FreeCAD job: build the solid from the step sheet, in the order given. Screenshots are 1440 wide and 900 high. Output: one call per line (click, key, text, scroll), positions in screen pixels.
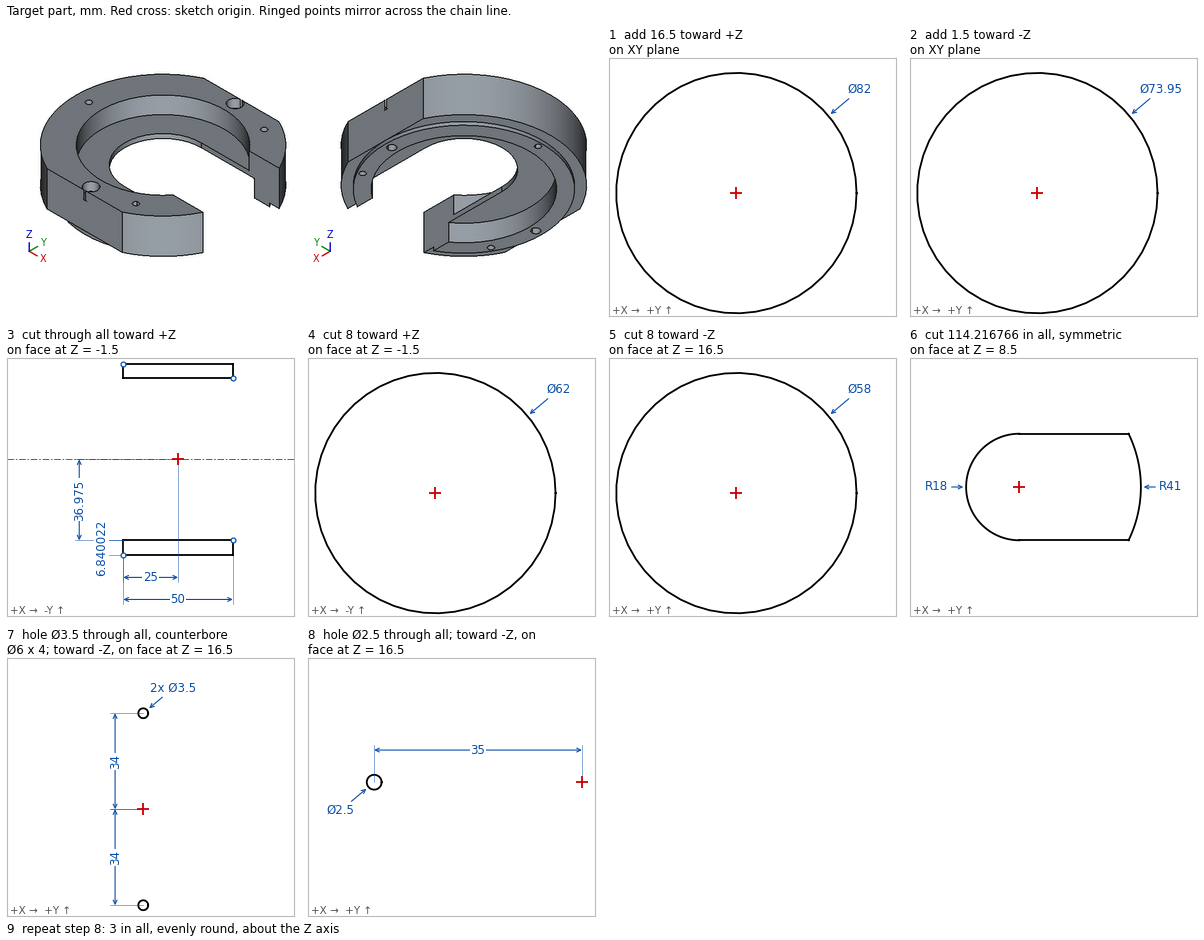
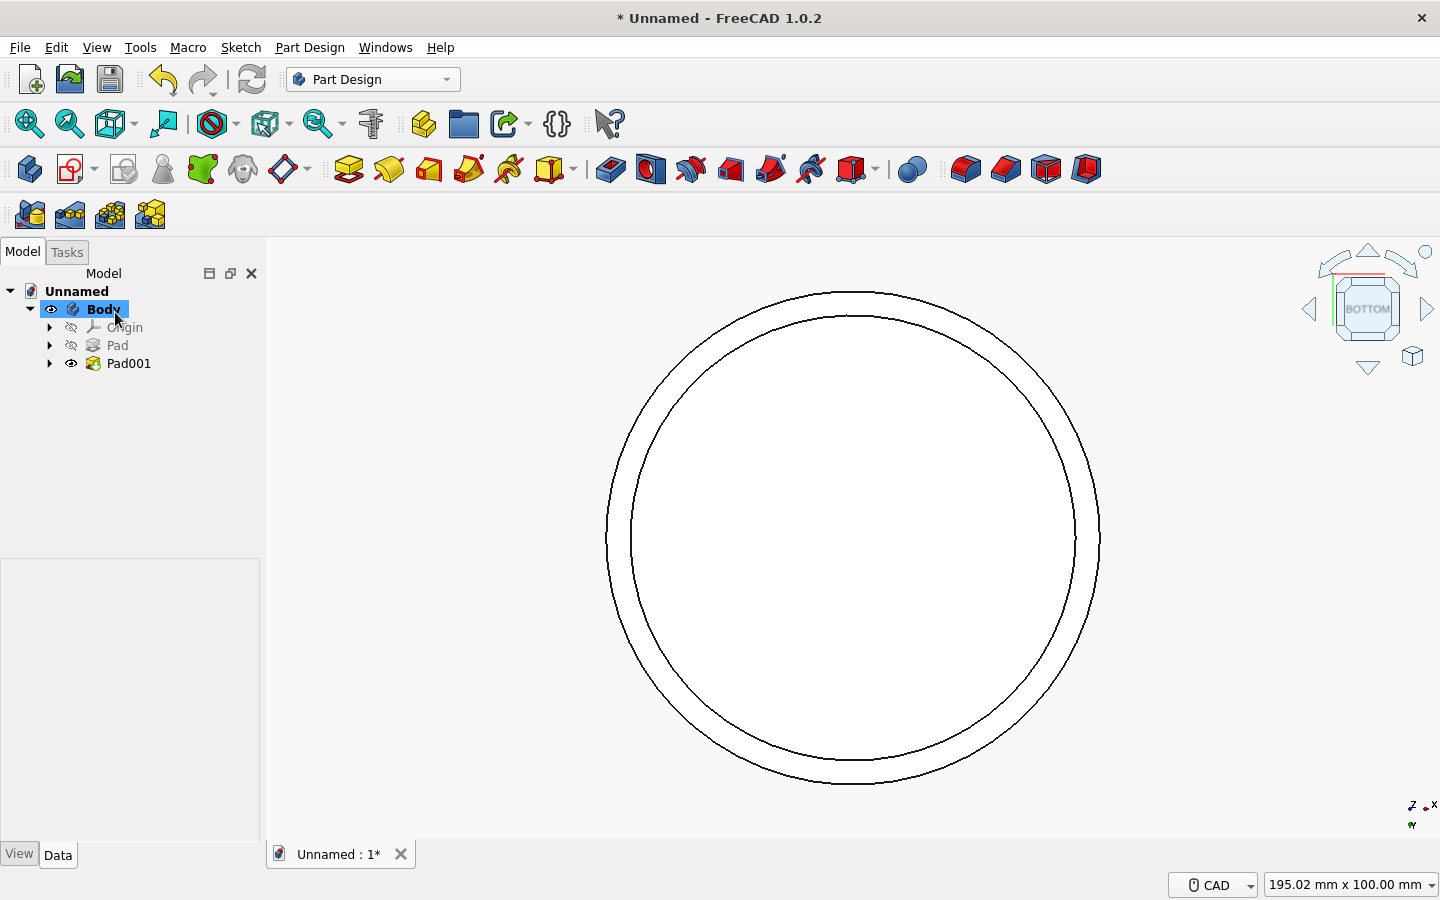
click(853, 537)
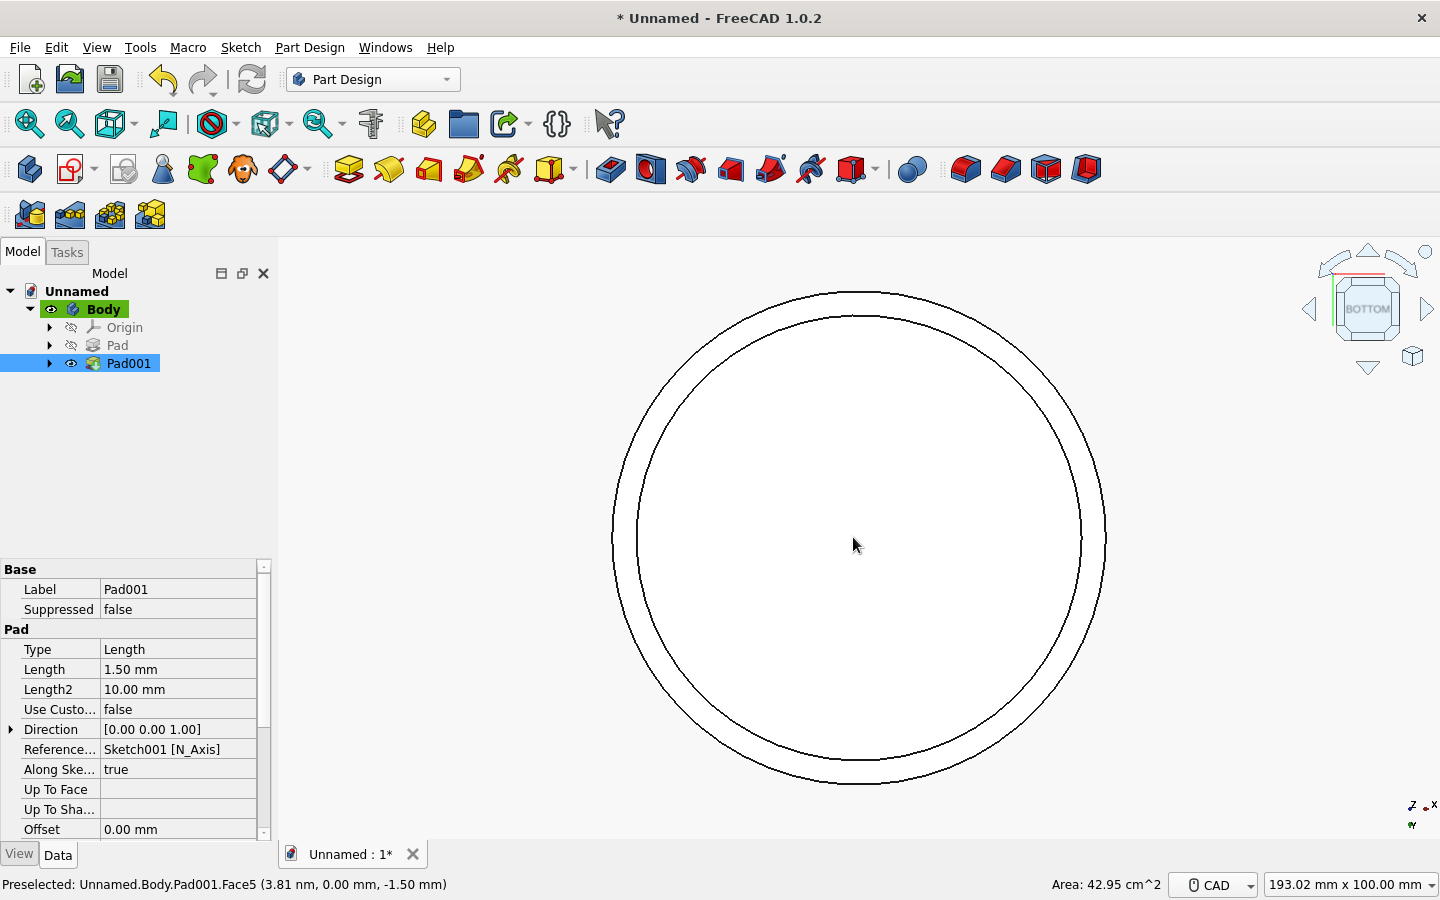
click(70, 170)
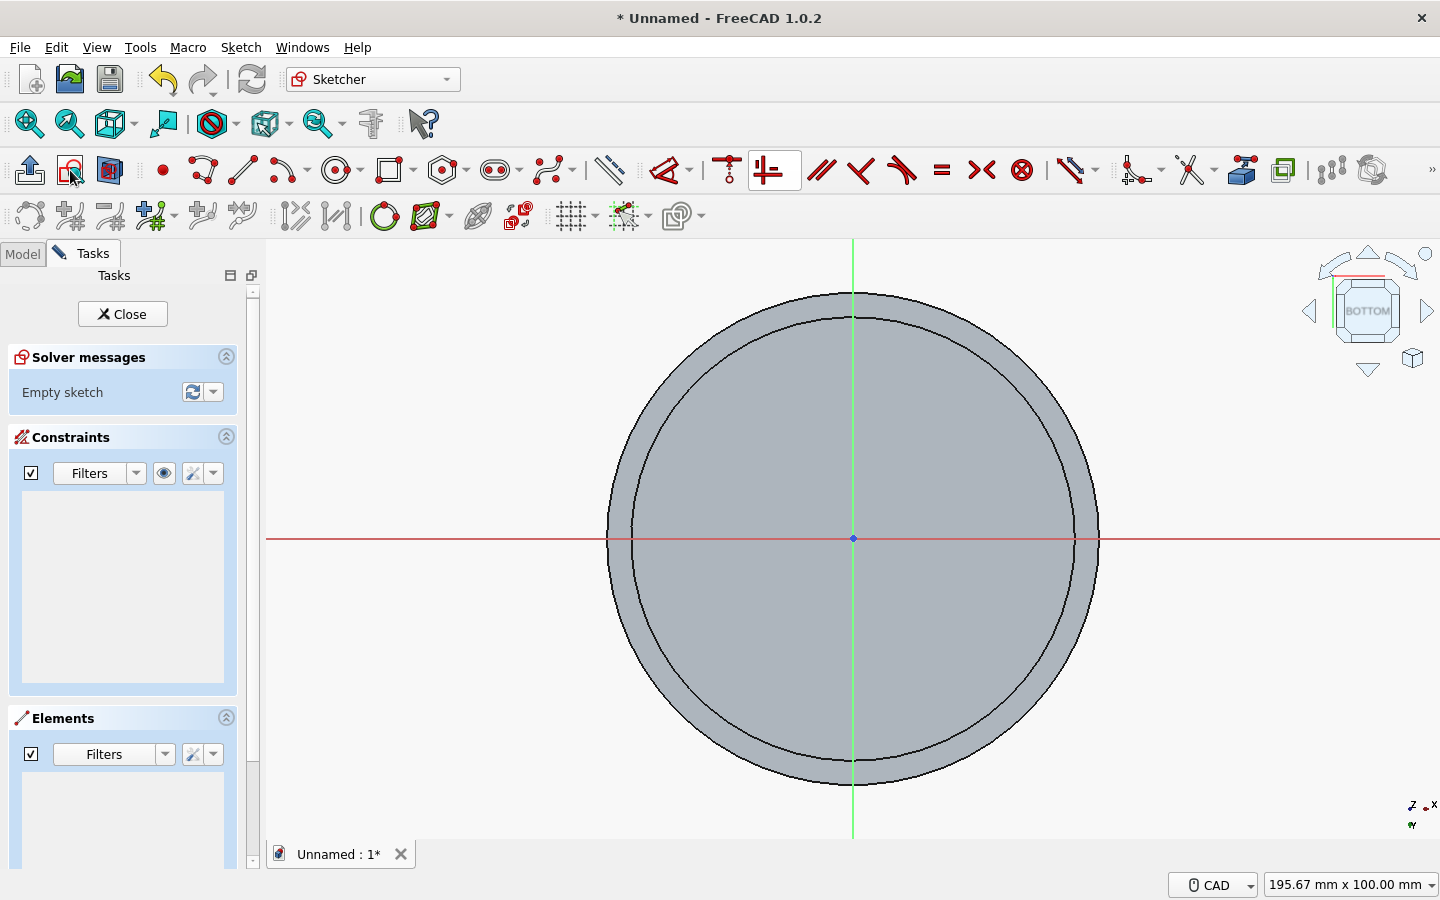
scroll(645, 539, down, 2)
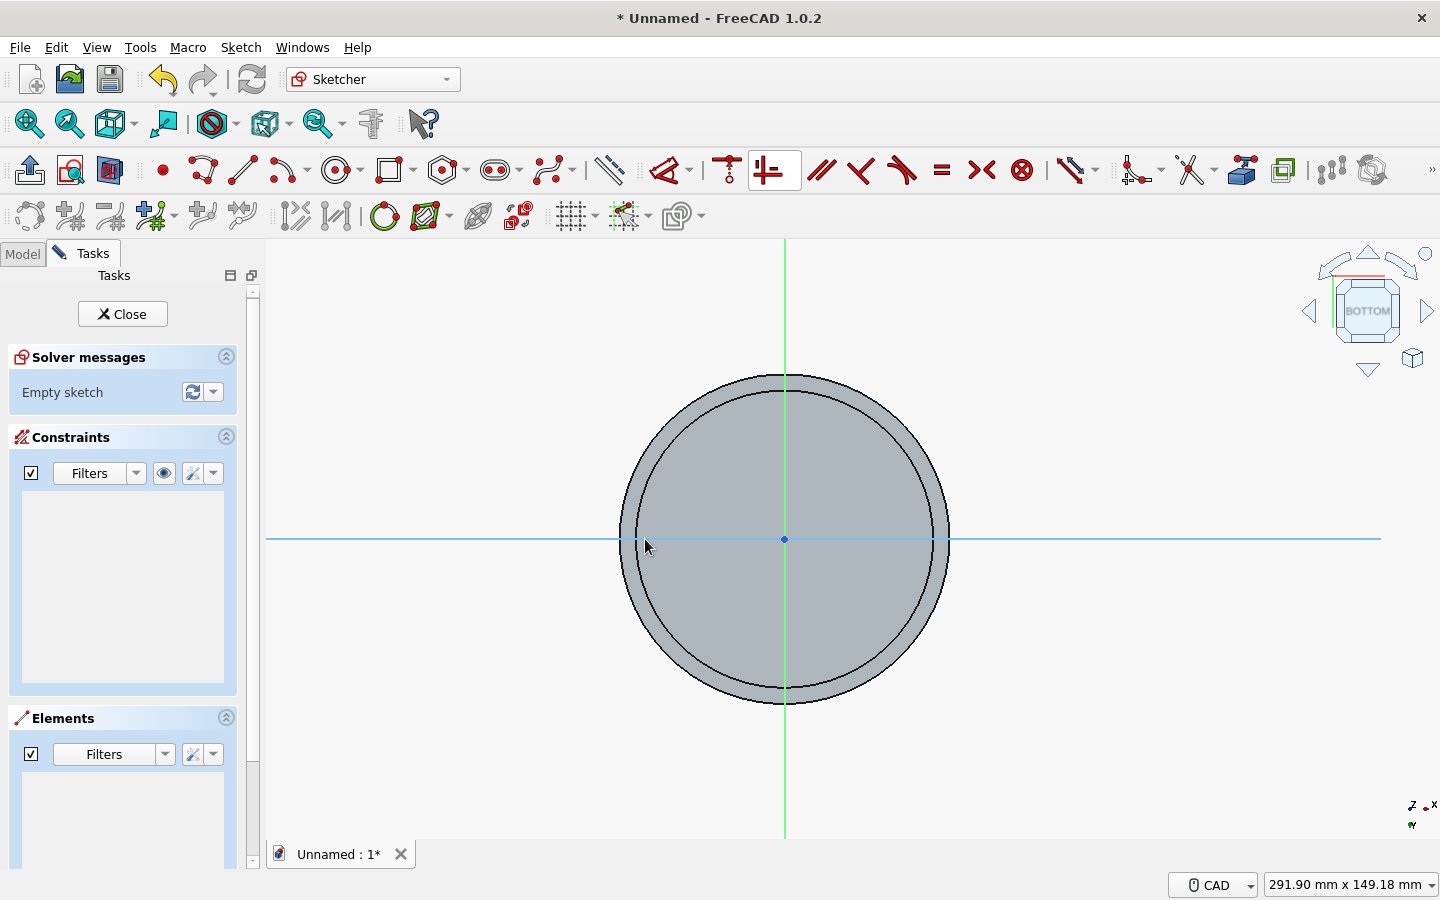
key(g)
key(r)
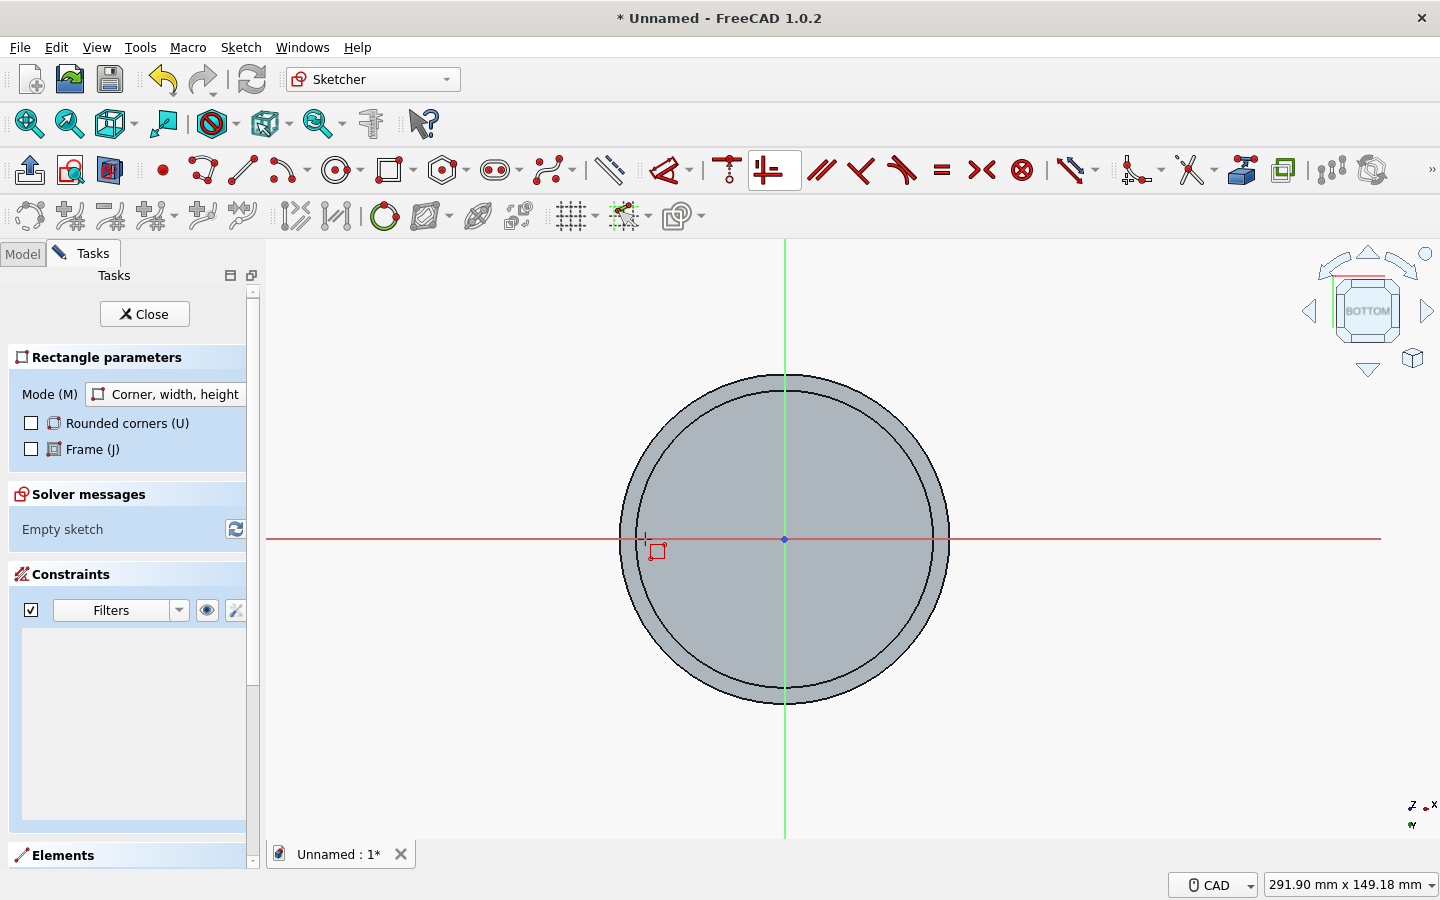
click(684, 688)
click(885, 715)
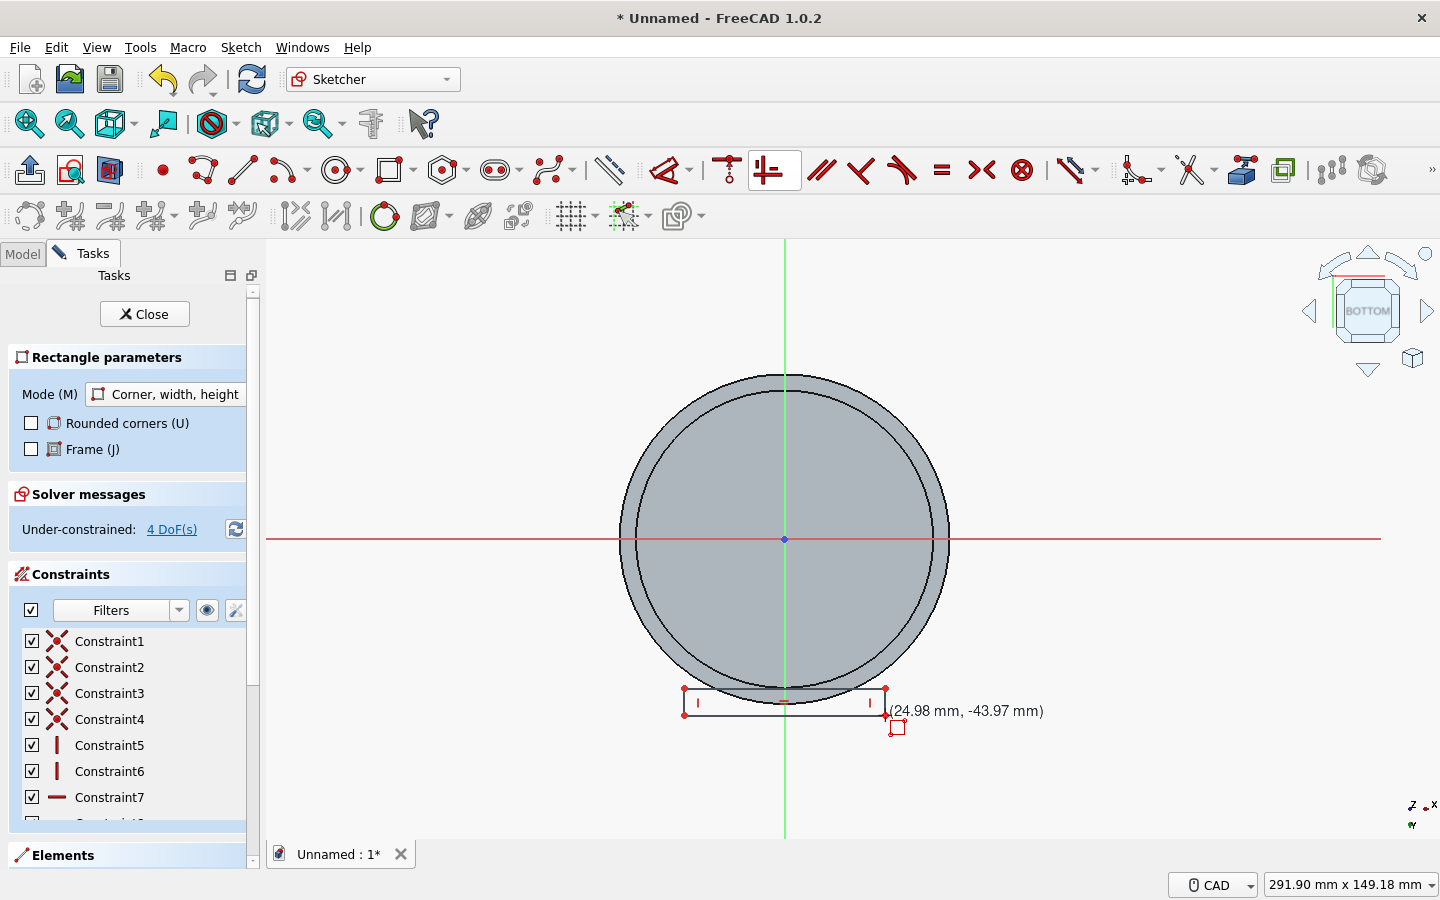
click(684, 363)
click(885, 390)
key(Escape)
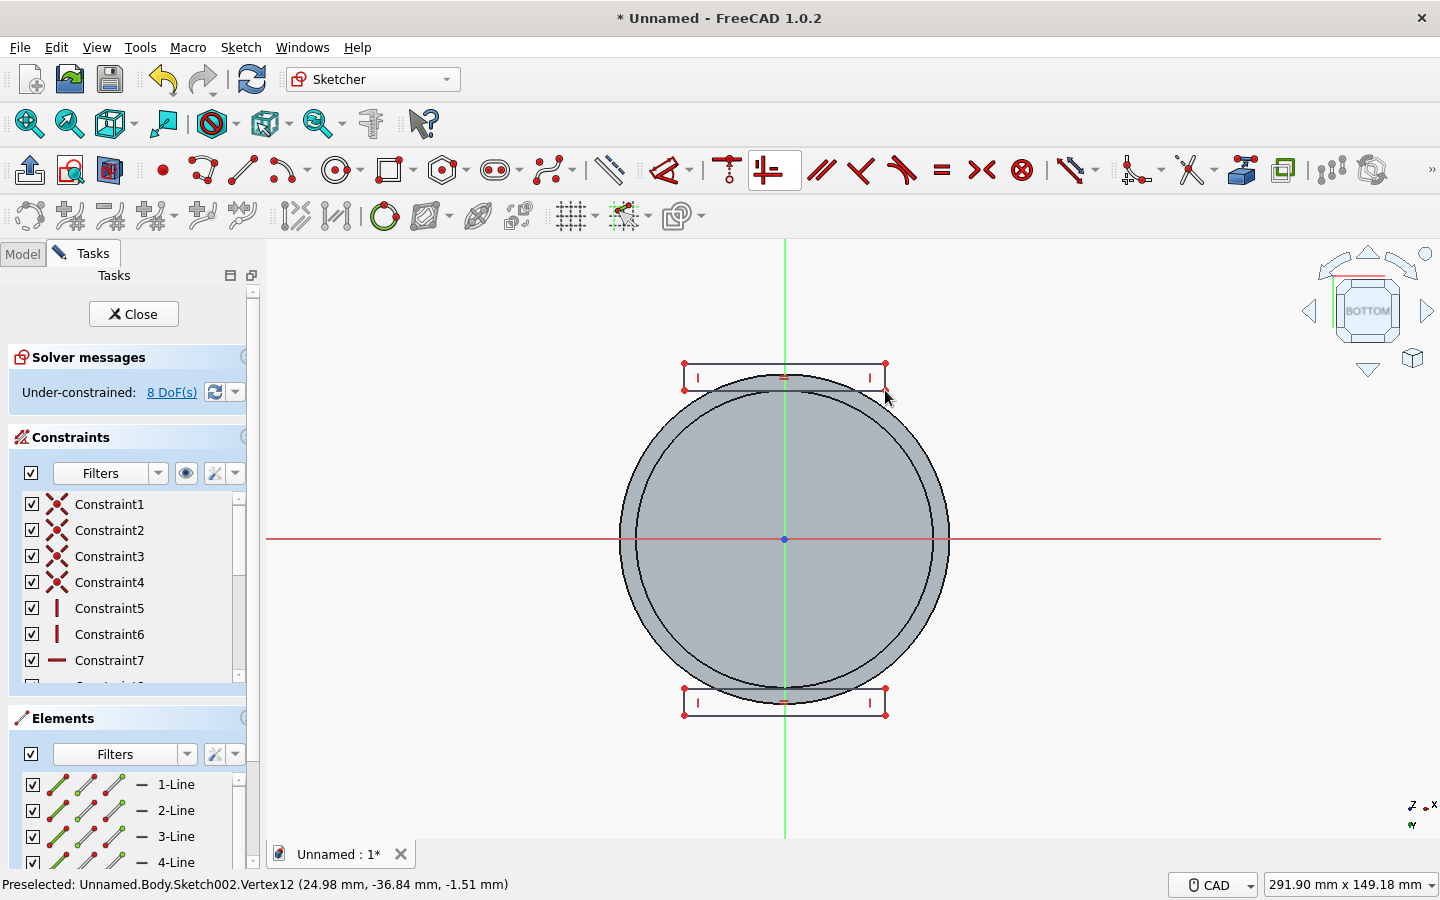
click(684, 716)